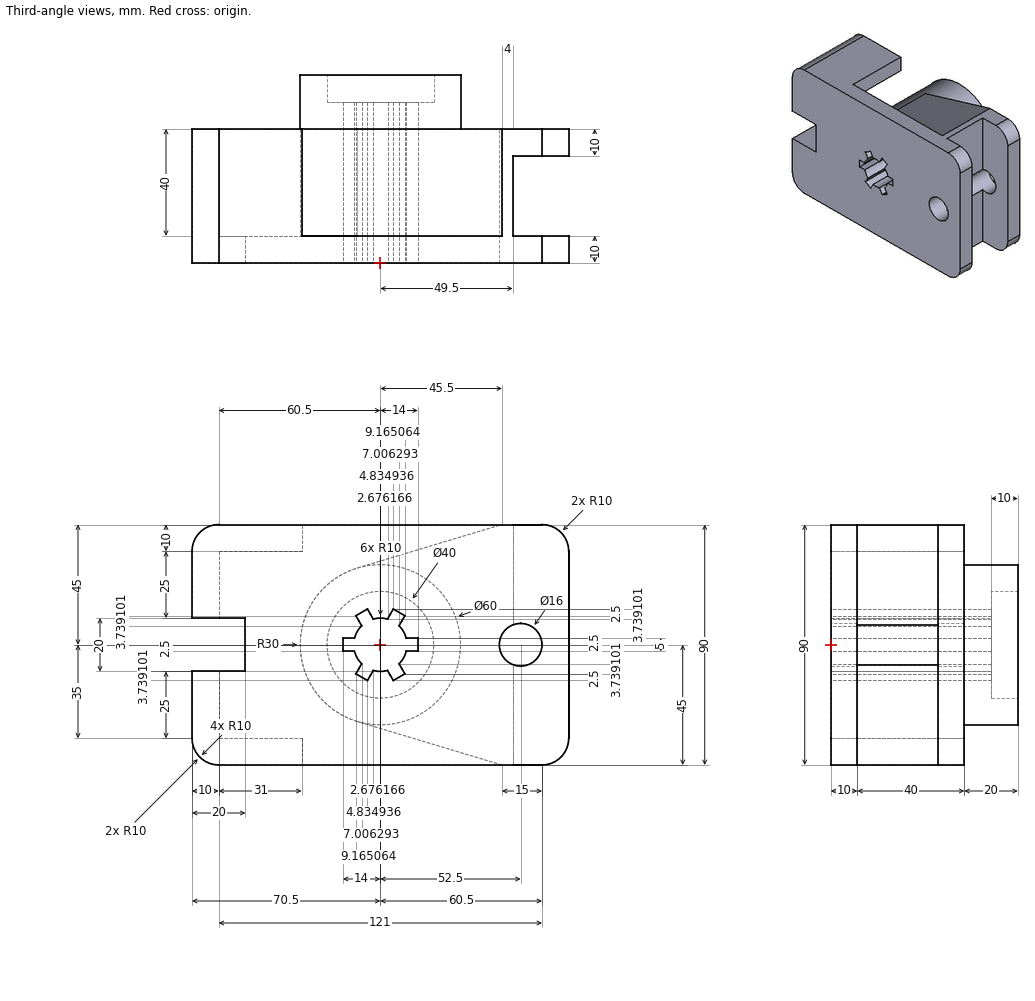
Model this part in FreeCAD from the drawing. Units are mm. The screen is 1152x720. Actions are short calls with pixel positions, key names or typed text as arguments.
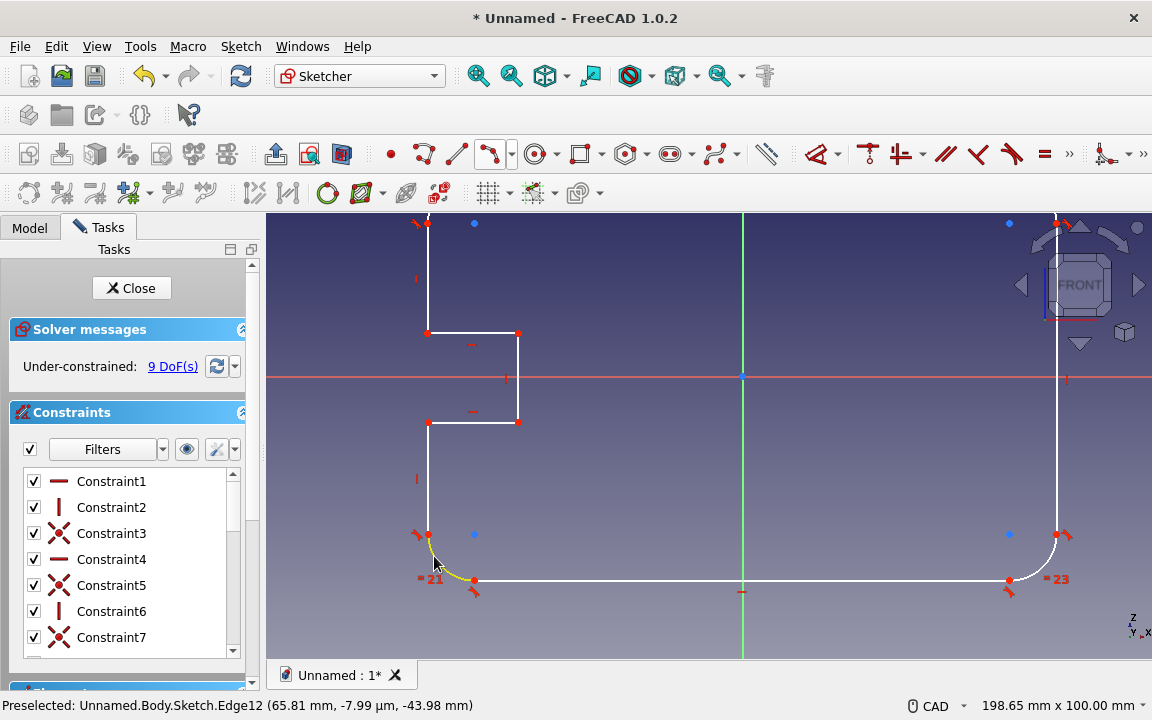
click(433, 555)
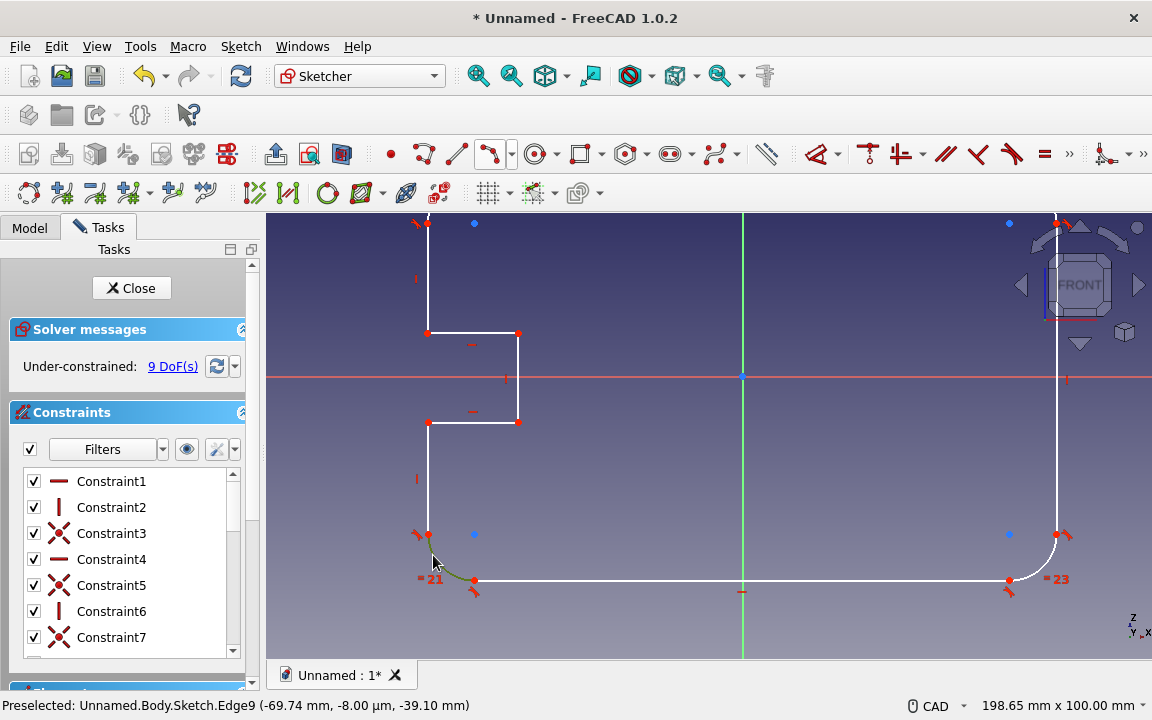
click(838, 154)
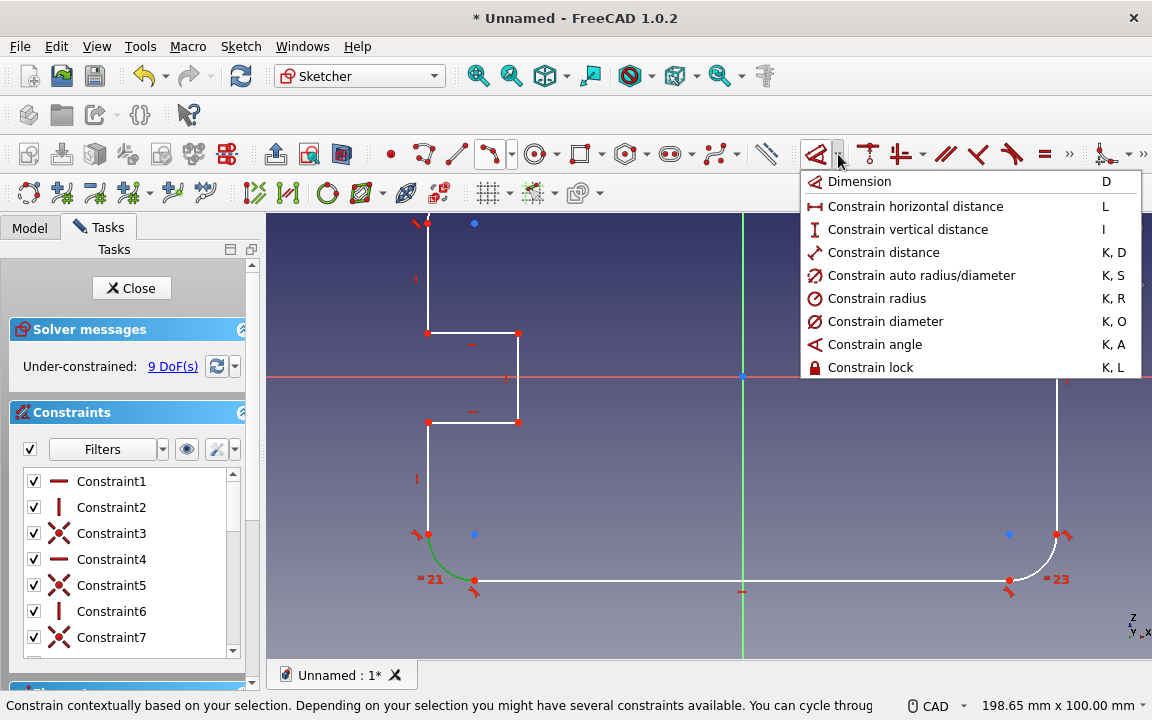
click(971, 298)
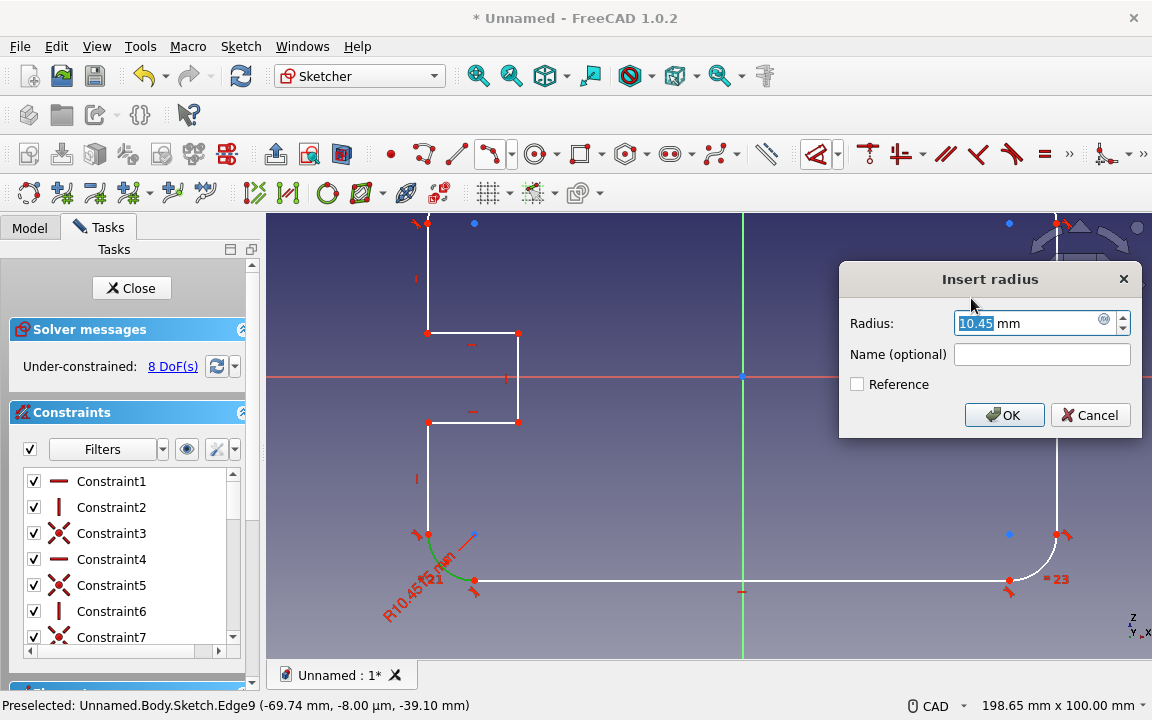
text(10)
key(Return)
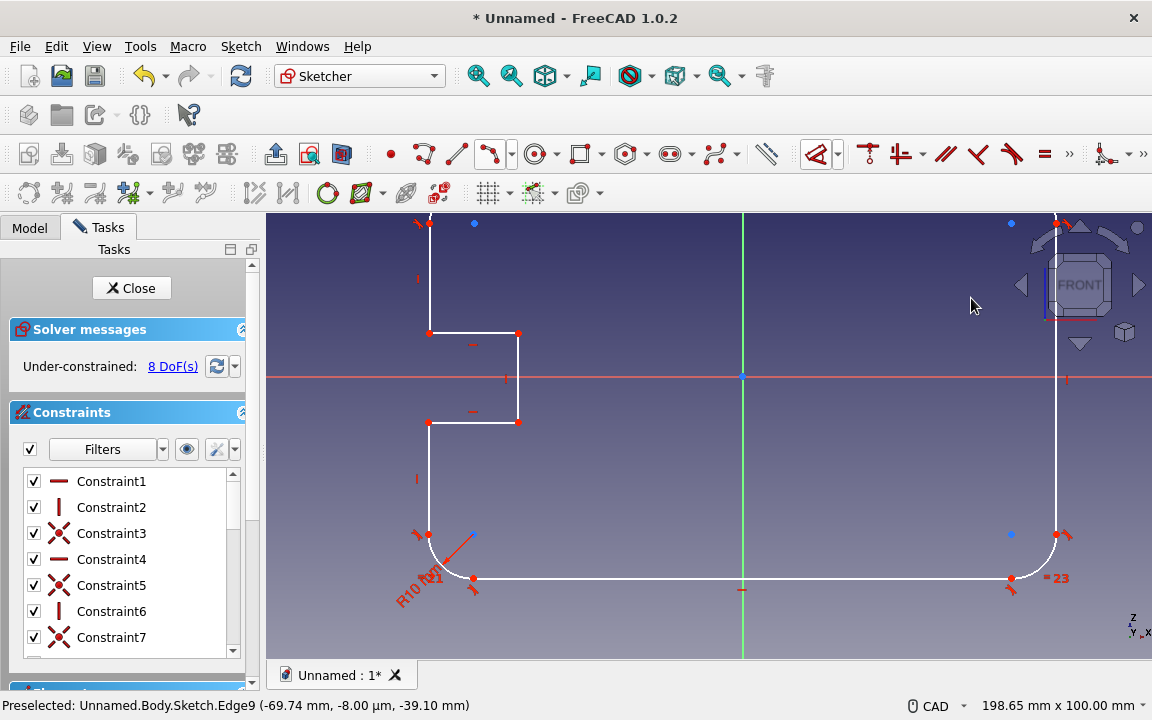
click(429, 501)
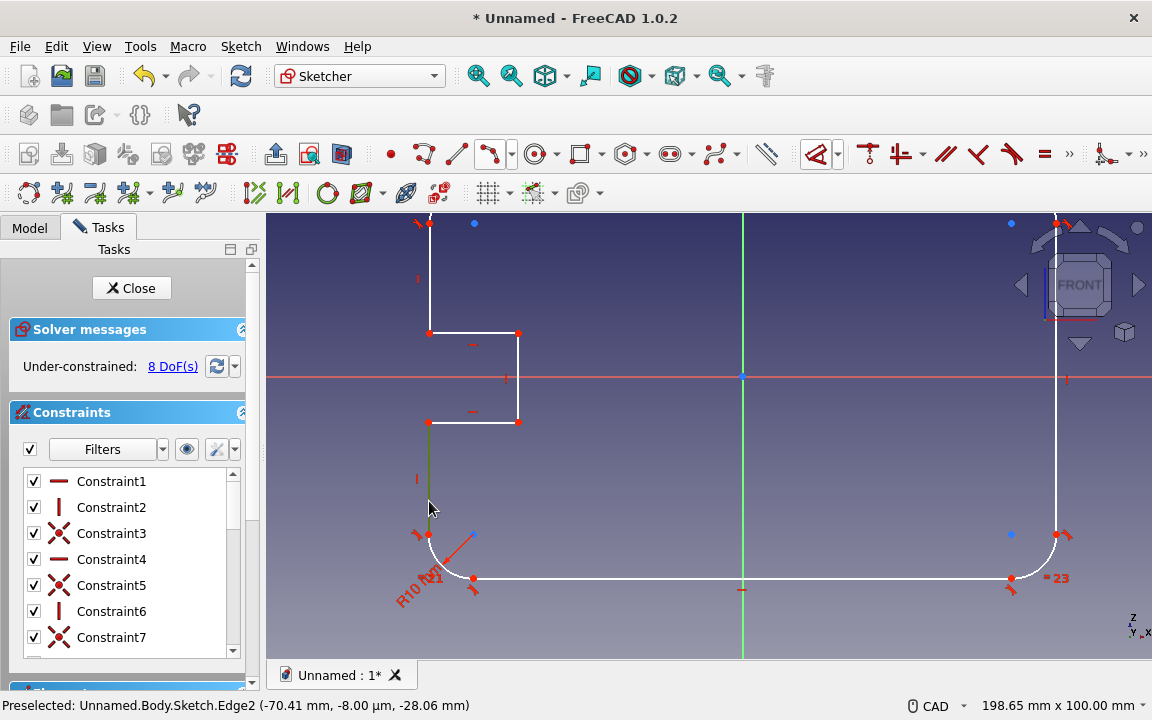
click(838, 154)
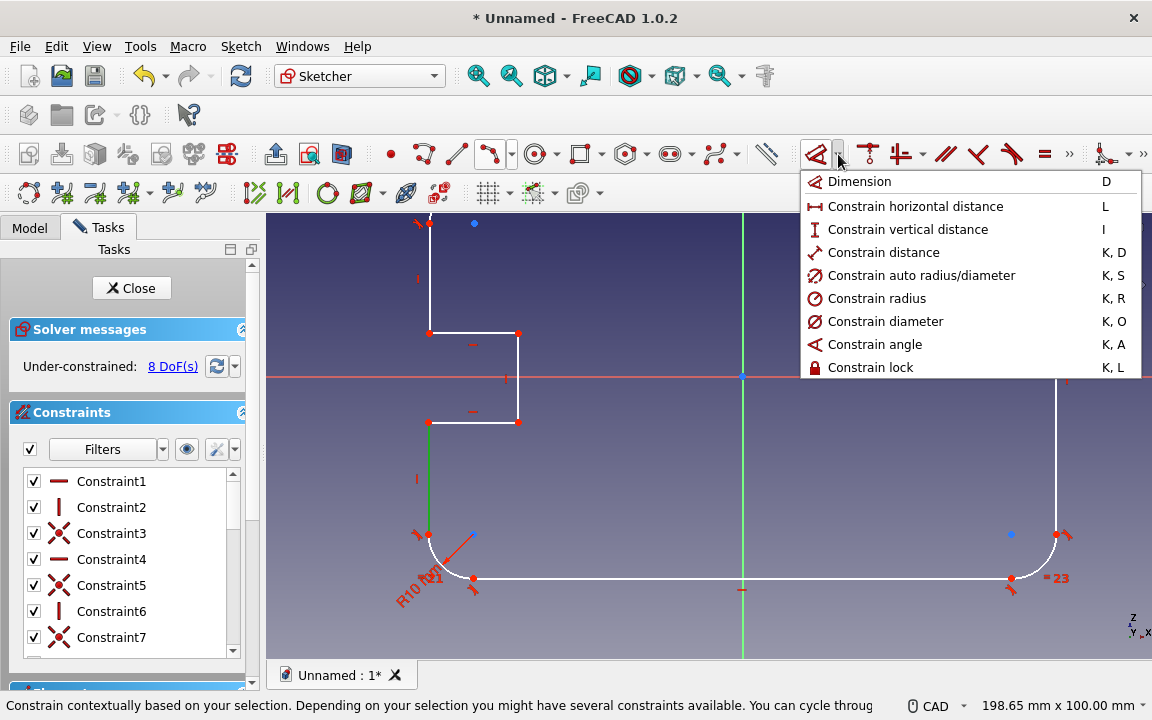
click(971, 230)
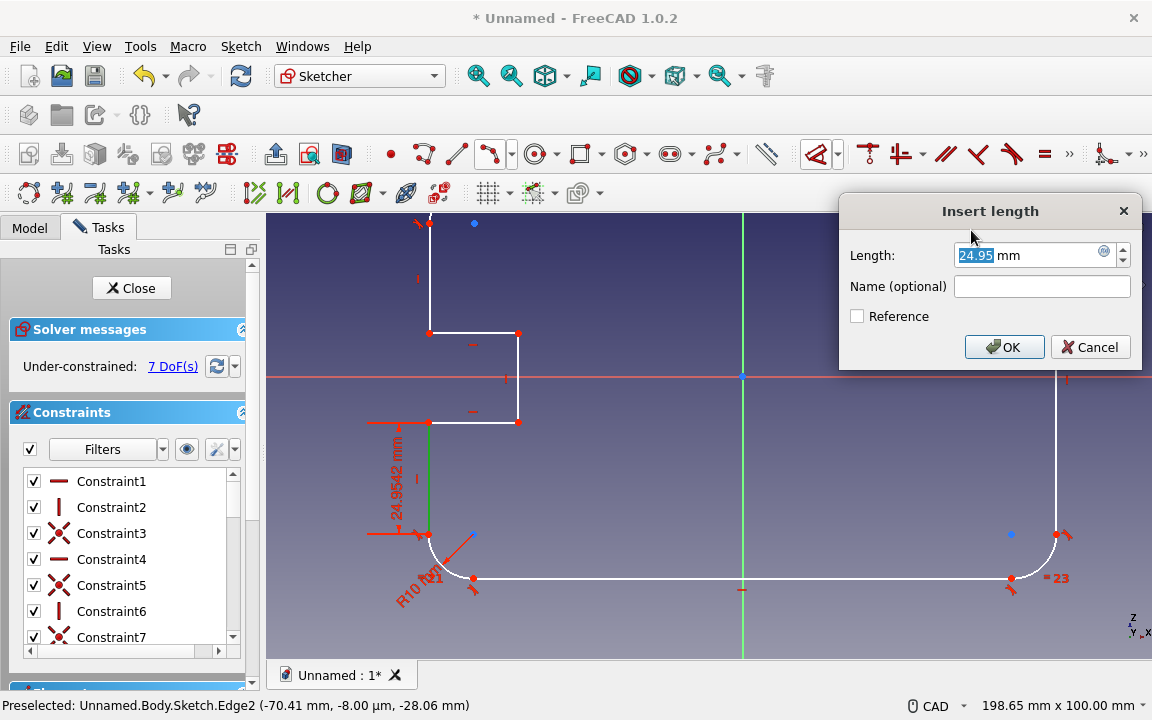
text(25)
key(Return)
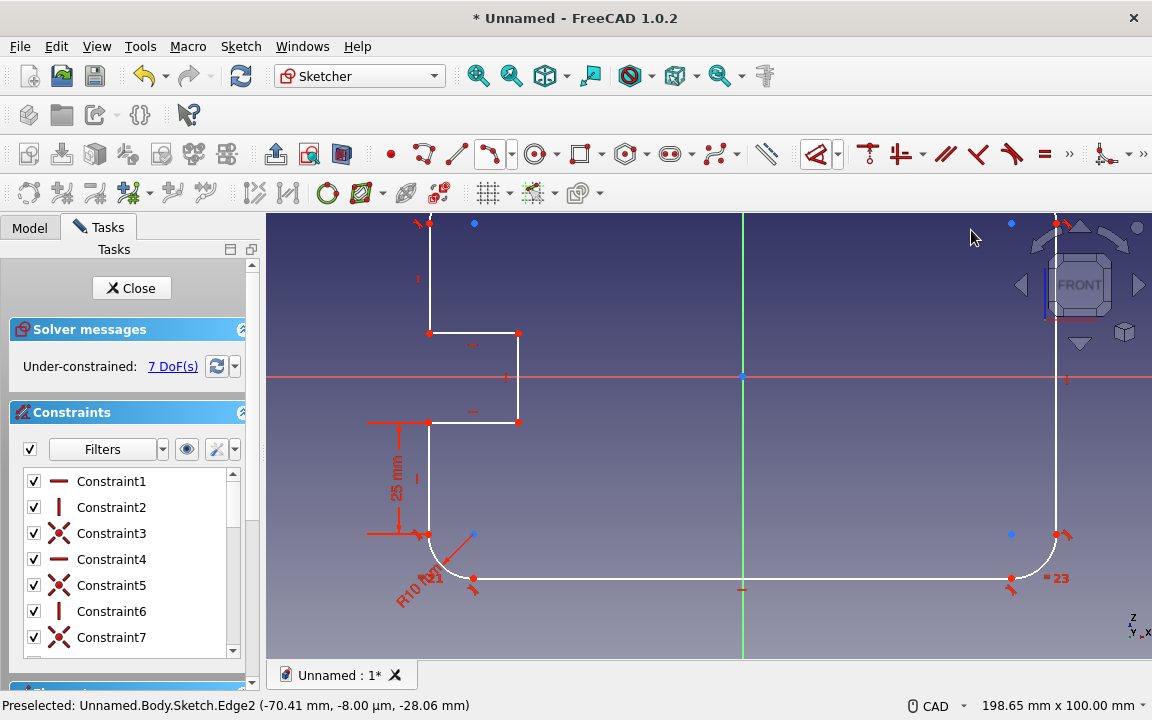
click(455, 423)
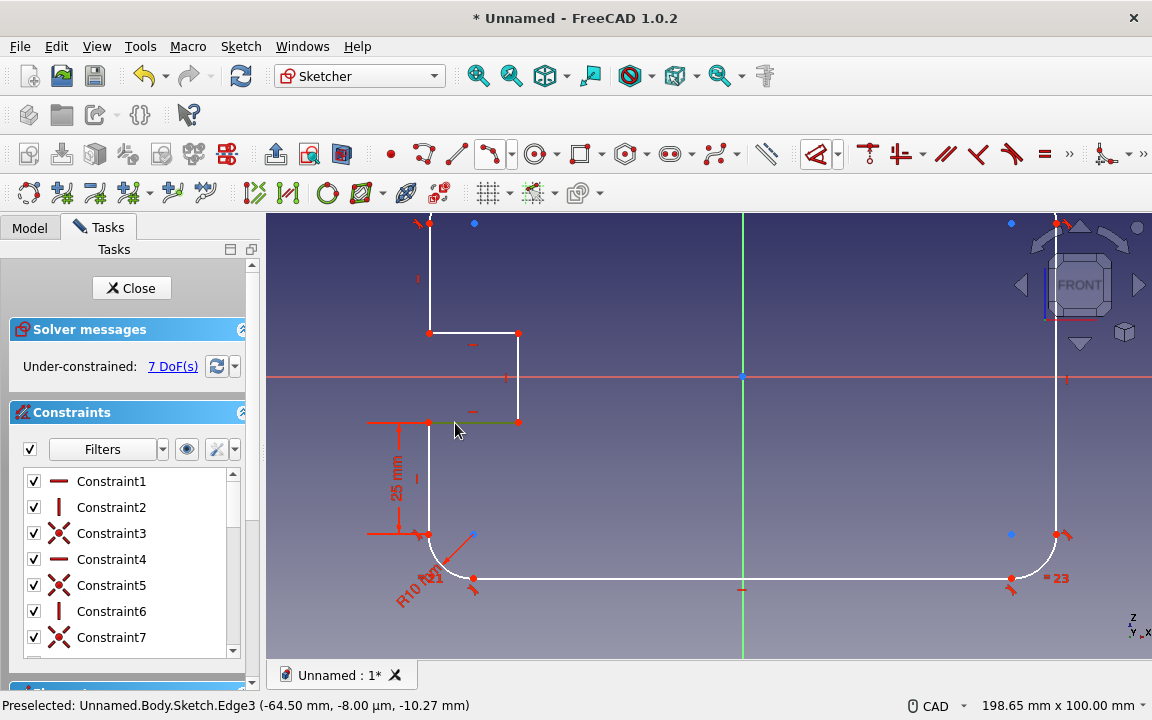
key(l)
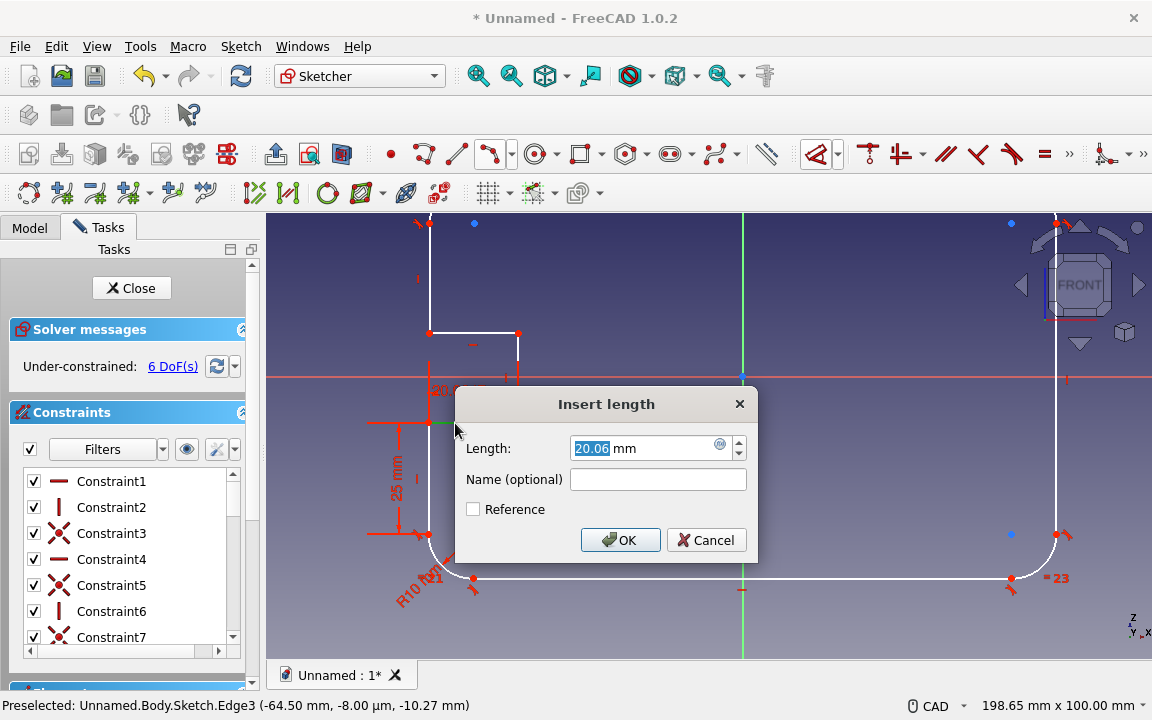
text(20)
key(Return)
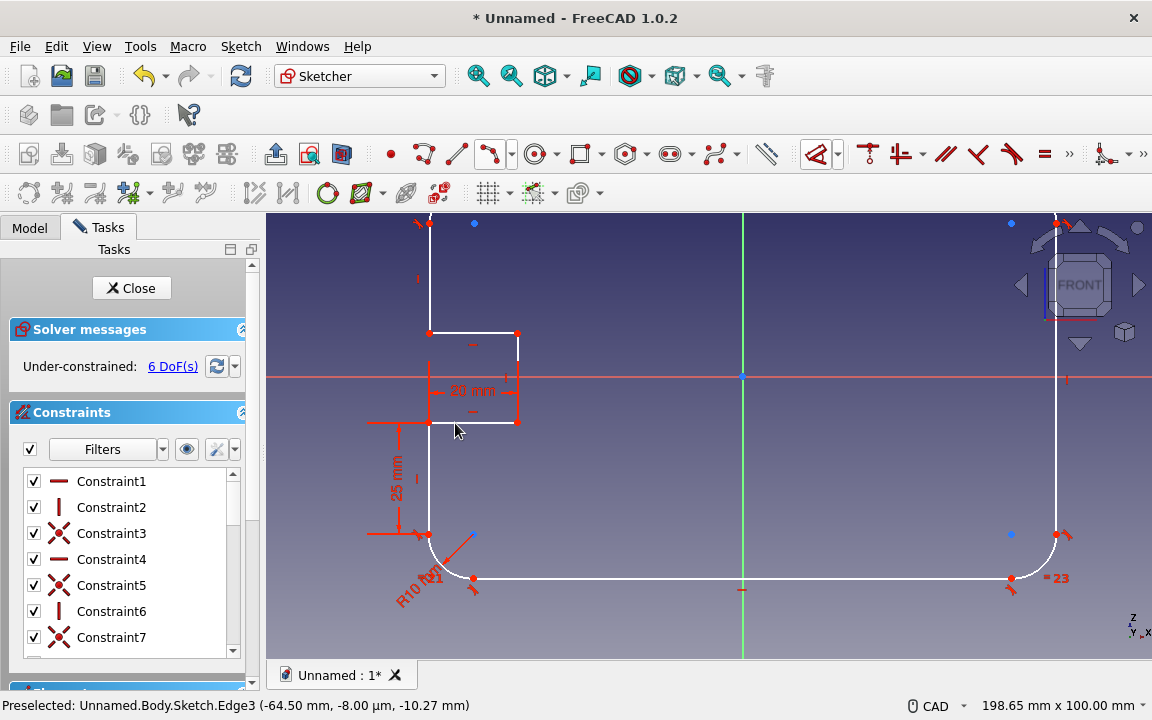
click(518, 396)